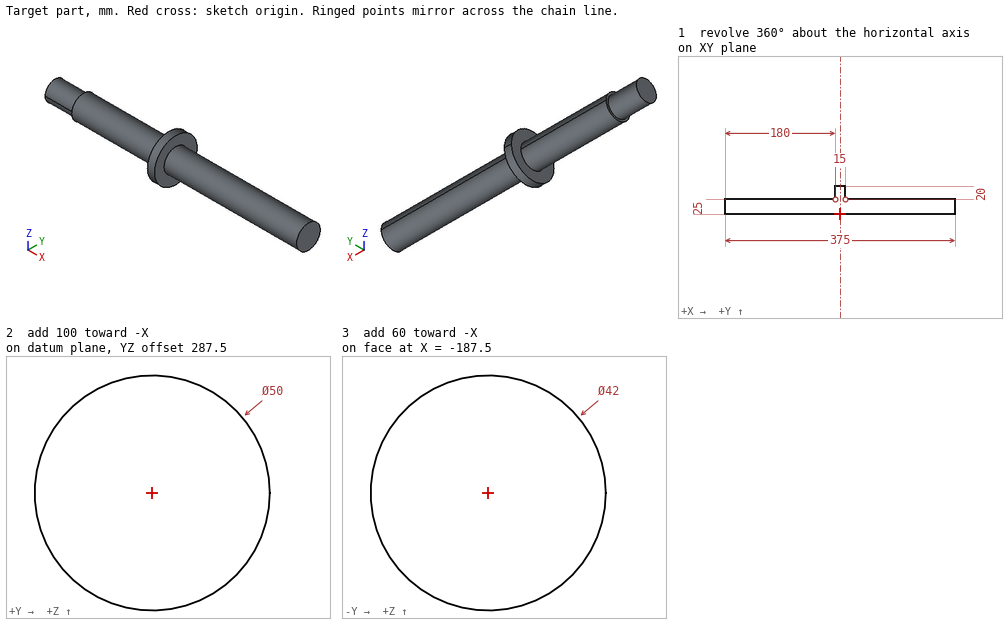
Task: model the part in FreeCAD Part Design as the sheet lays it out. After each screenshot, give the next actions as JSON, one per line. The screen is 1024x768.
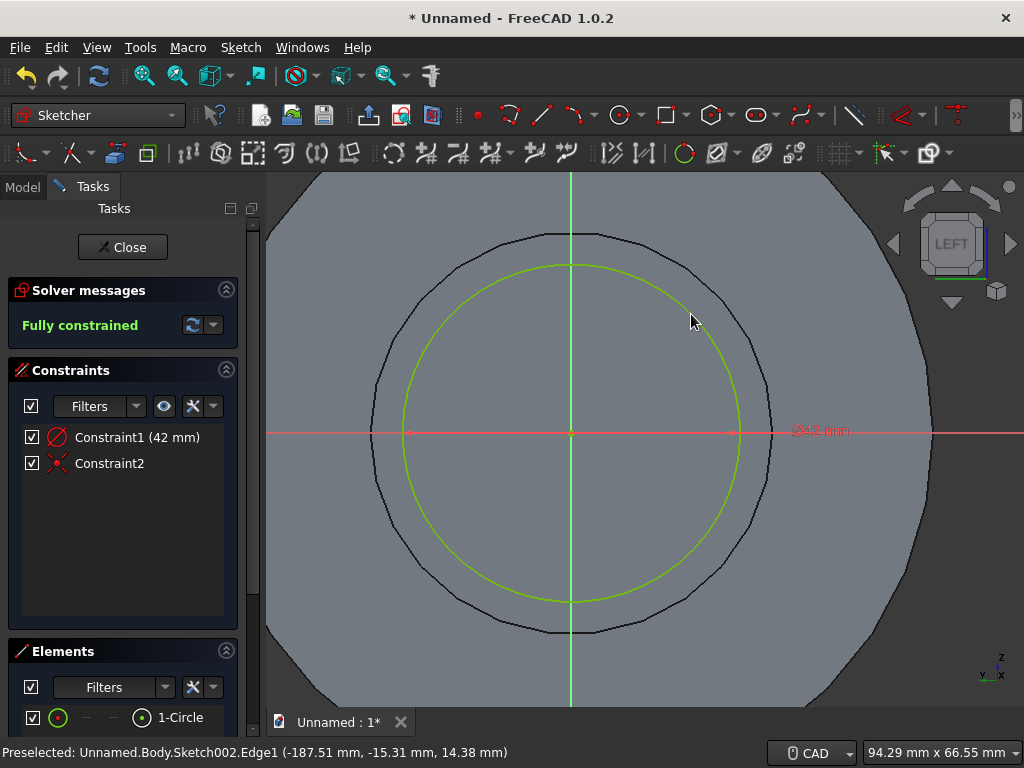
{"action": "left_click", "coordinate": [123, 247]}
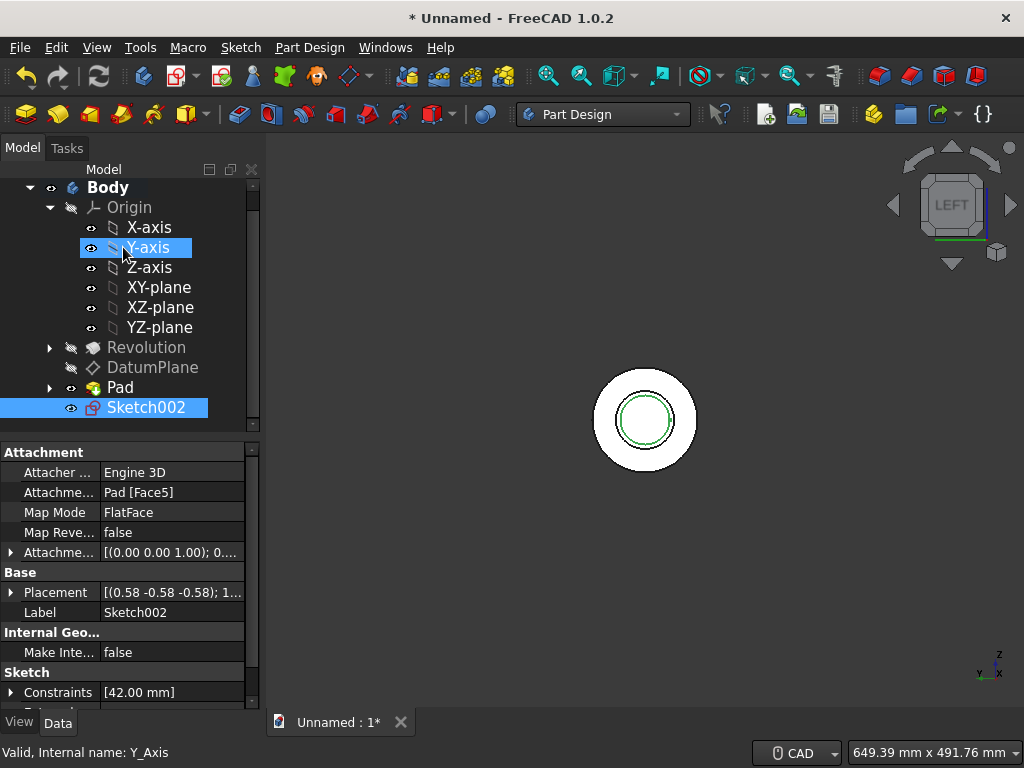
{"action": "left_click", "coordinate": [26, 114]}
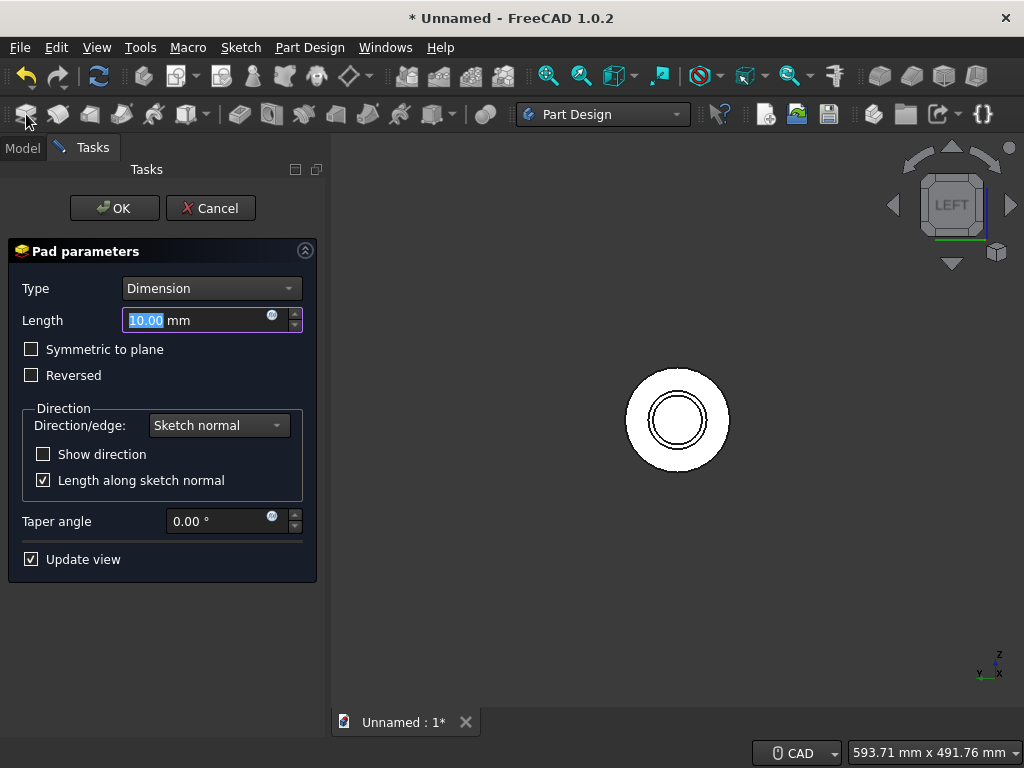
{"action": "type", "text": "60"}
{"action": "key", "text": "Tab"}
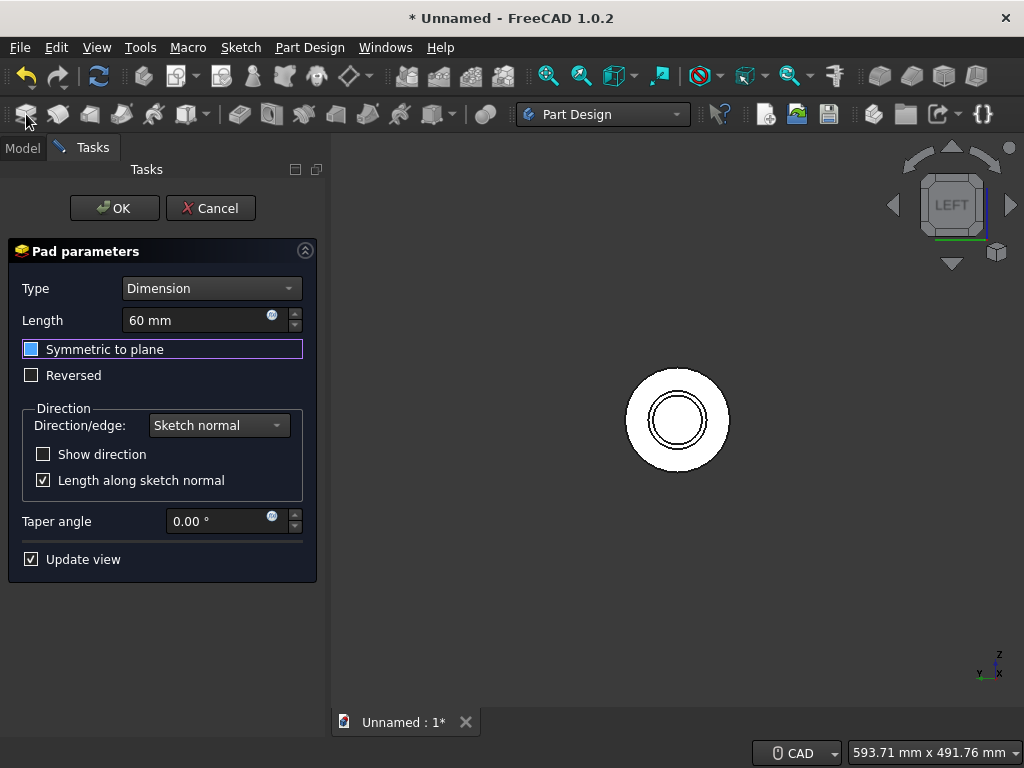
{"action": "left_click", "coordinate": [115, 208]}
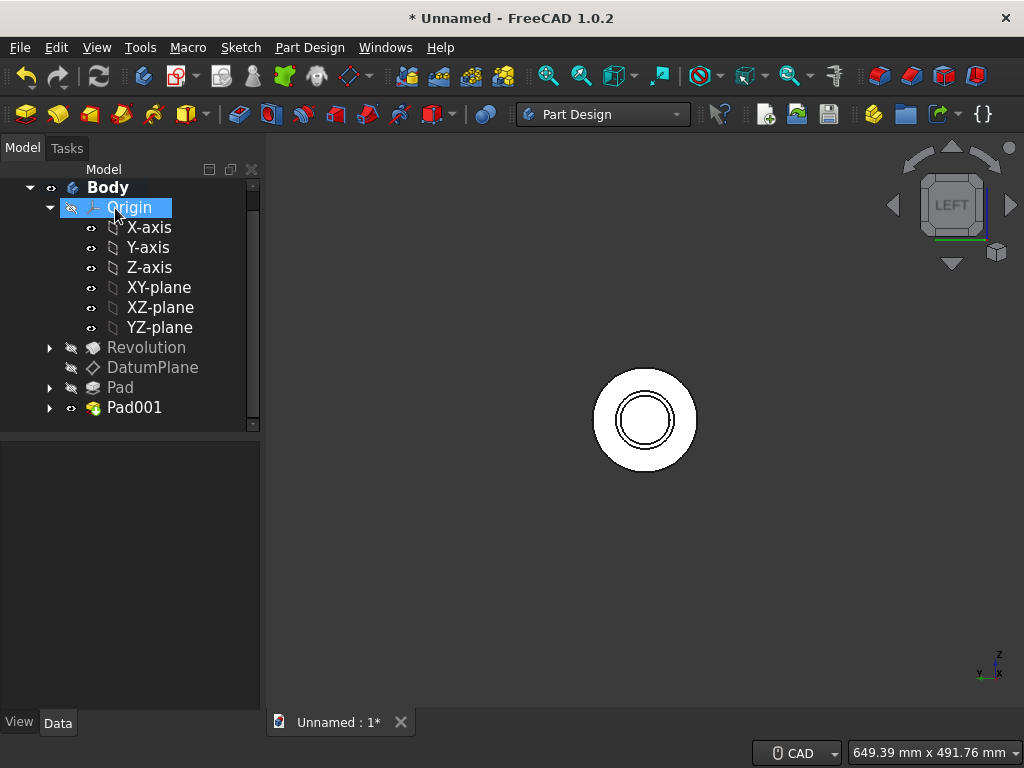
{"action": "key", "text": "0"}